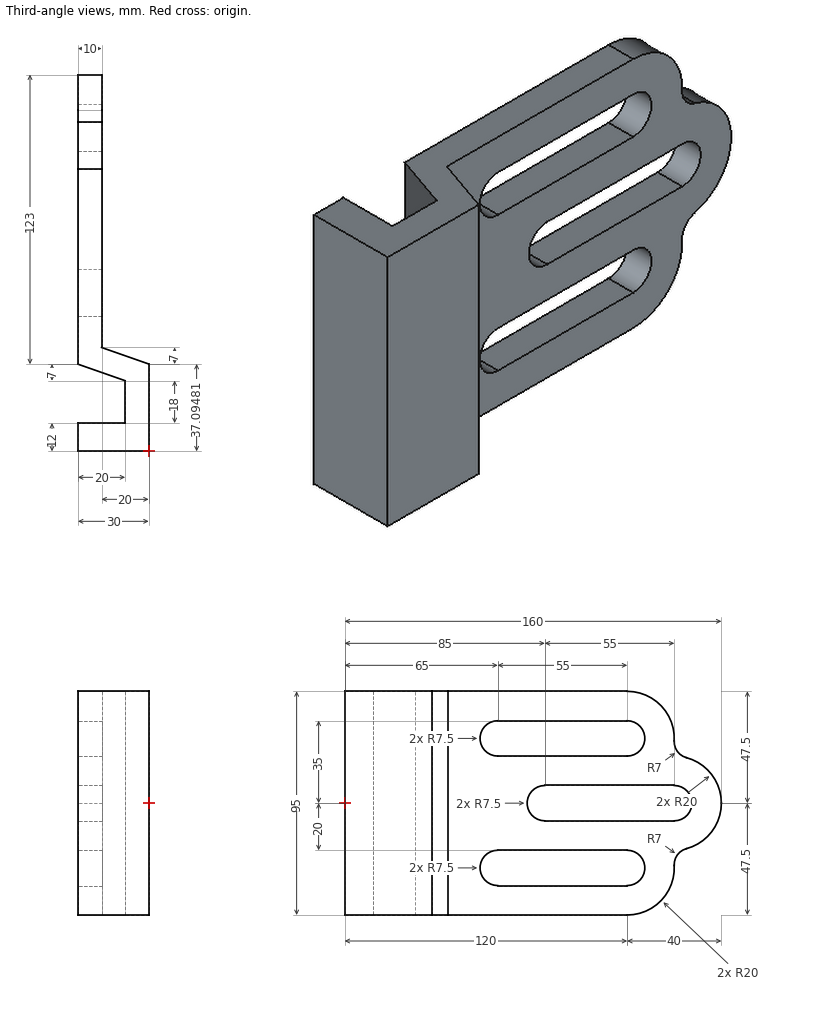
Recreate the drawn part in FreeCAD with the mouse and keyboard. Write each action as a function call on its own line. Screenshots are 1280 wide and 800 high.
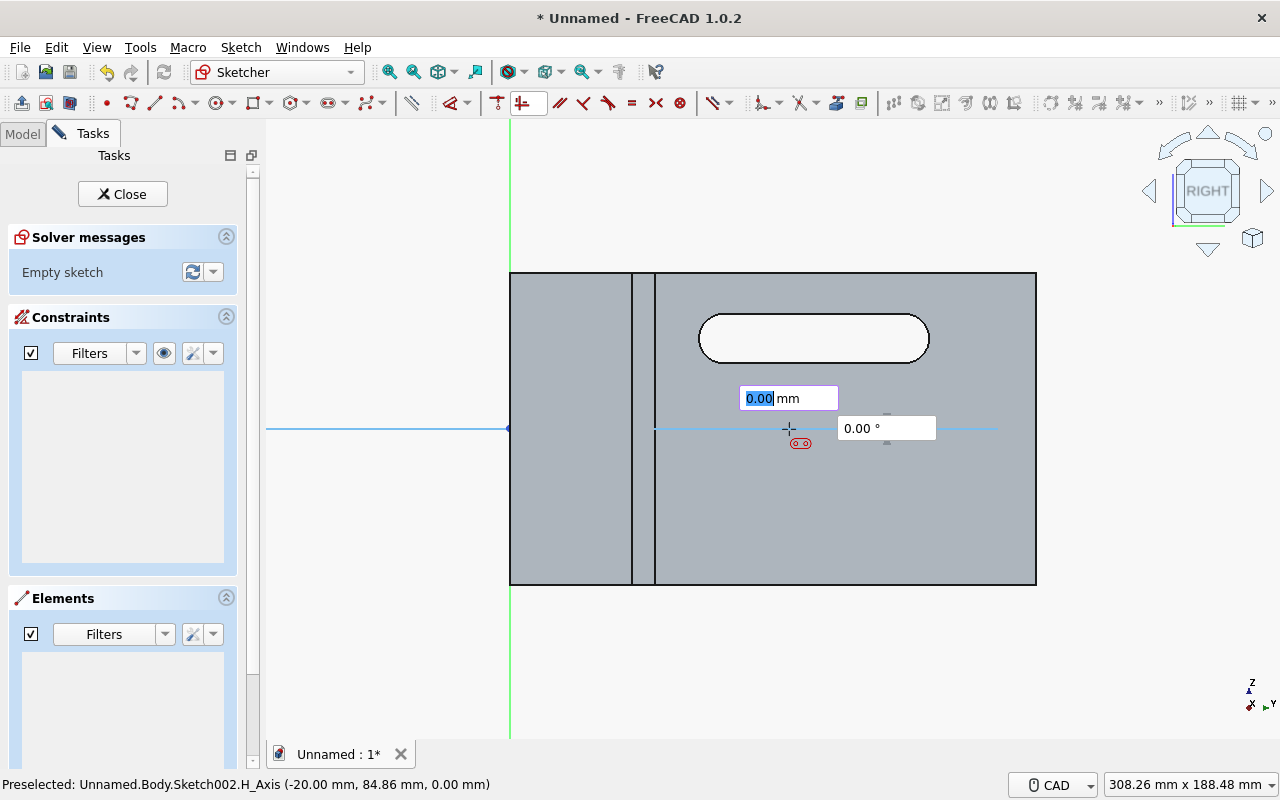
click(970, 420)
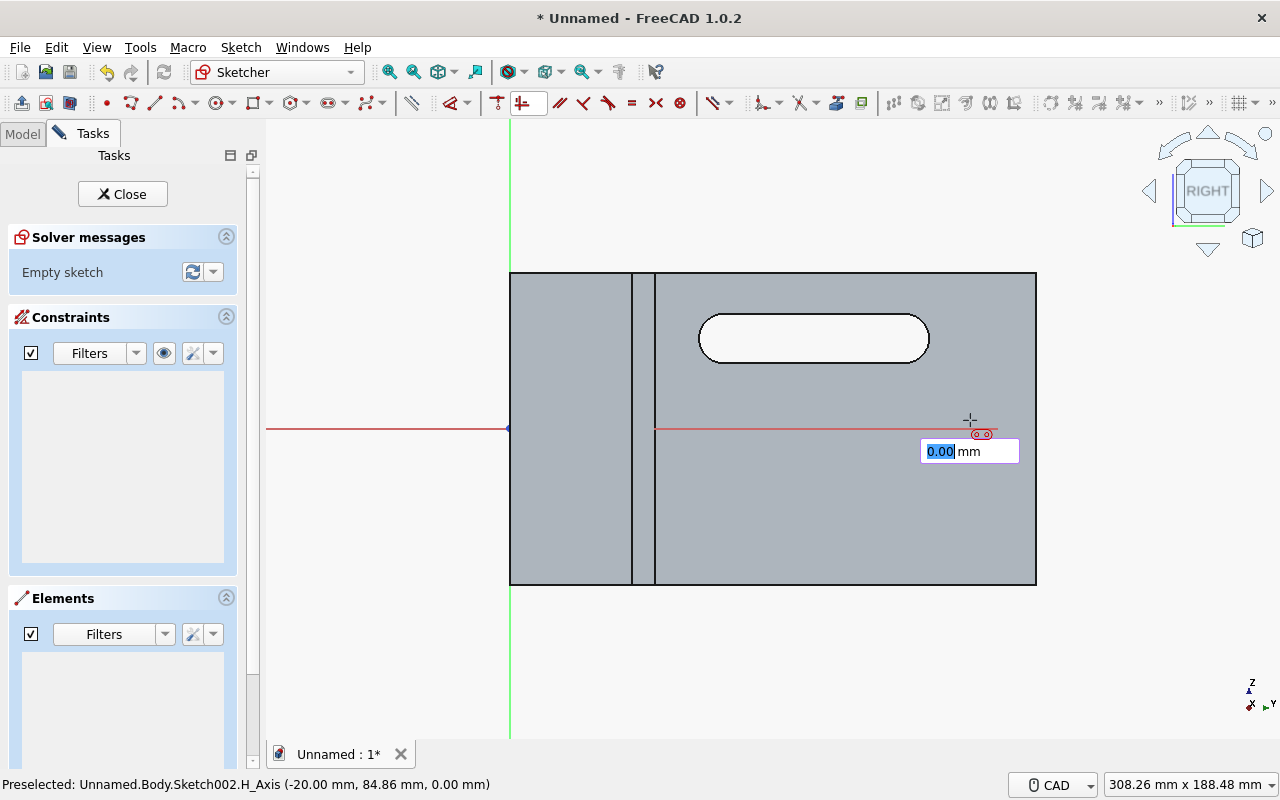
click(880, 404)
key(Escape)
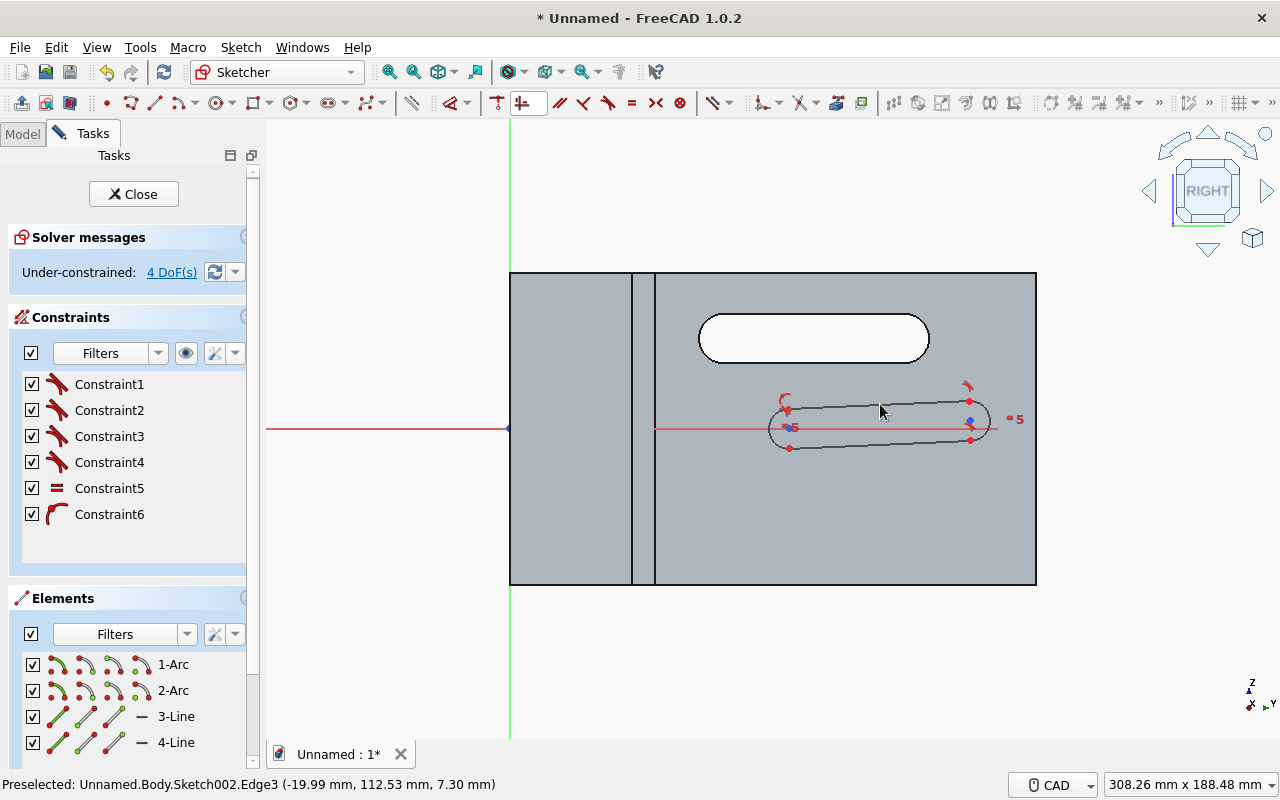
click(842, 407)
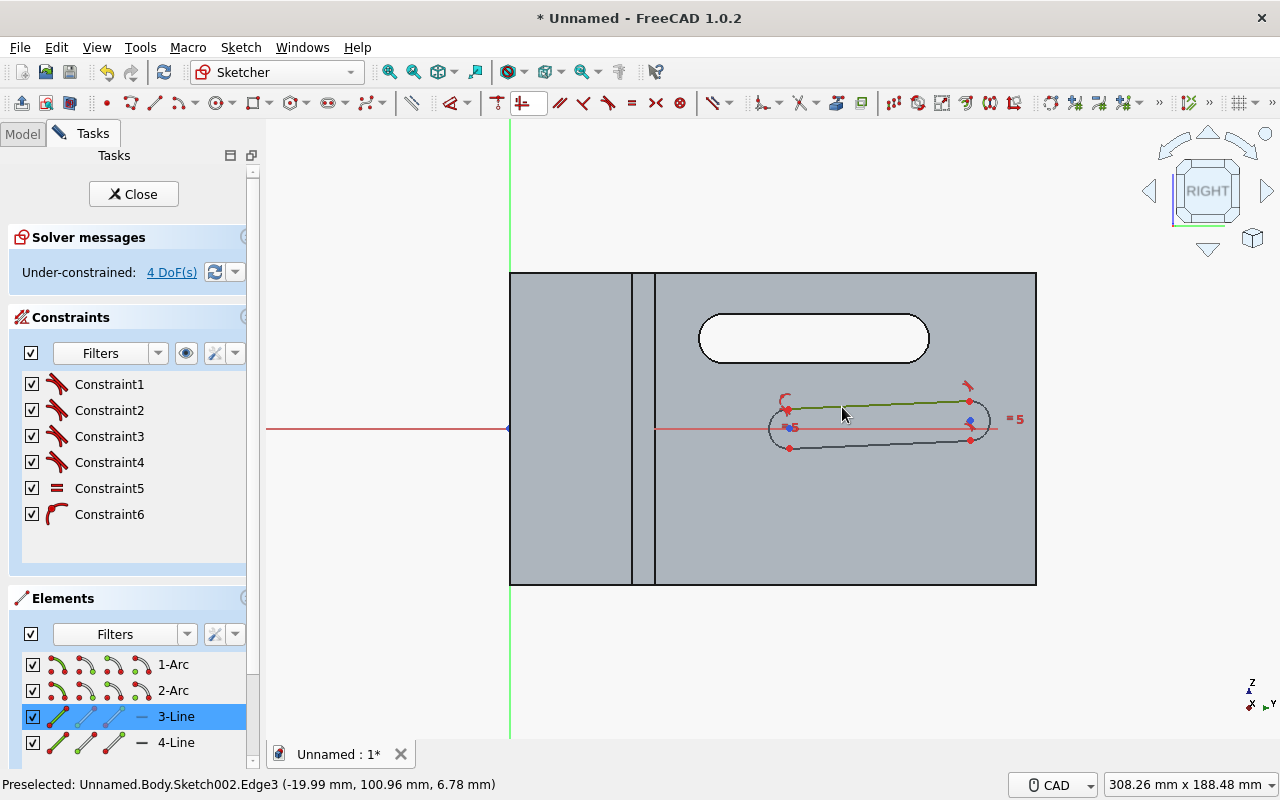
click(542, 104)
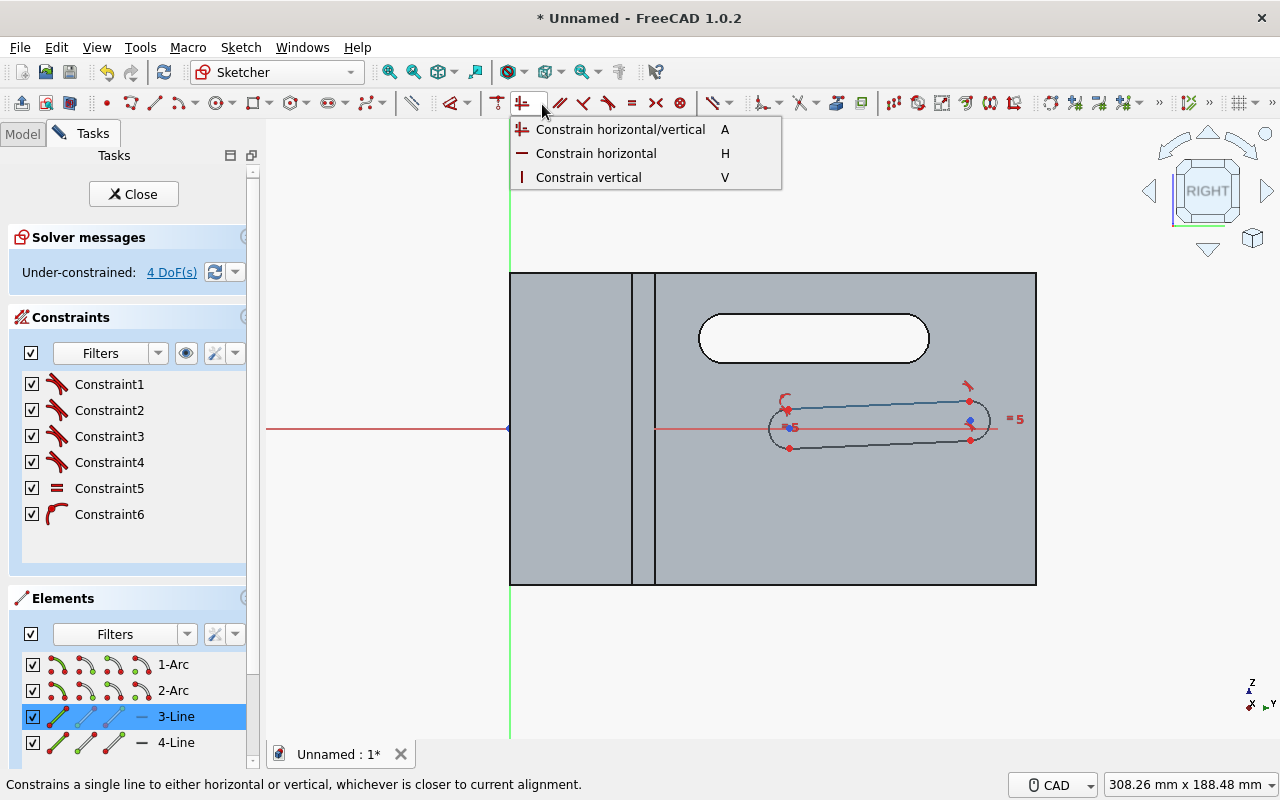
click(646, 153)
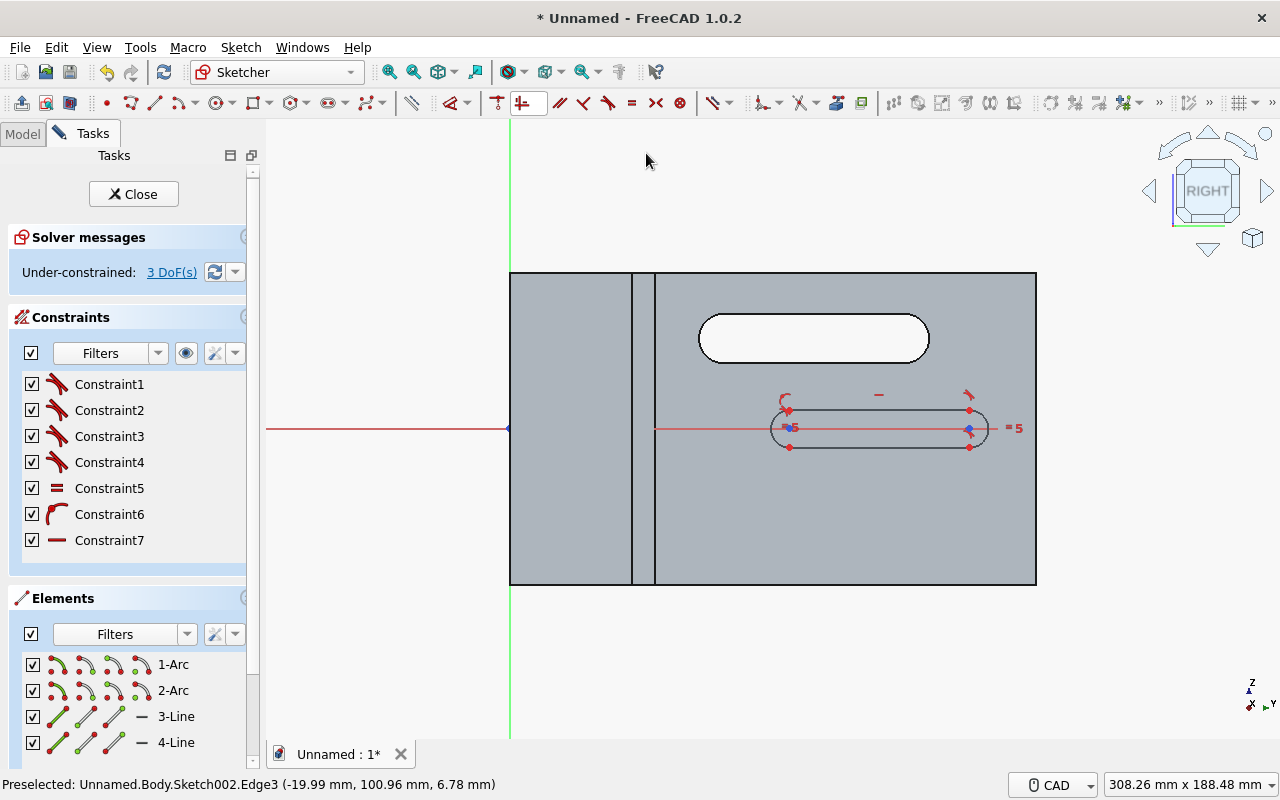
click(450, 104)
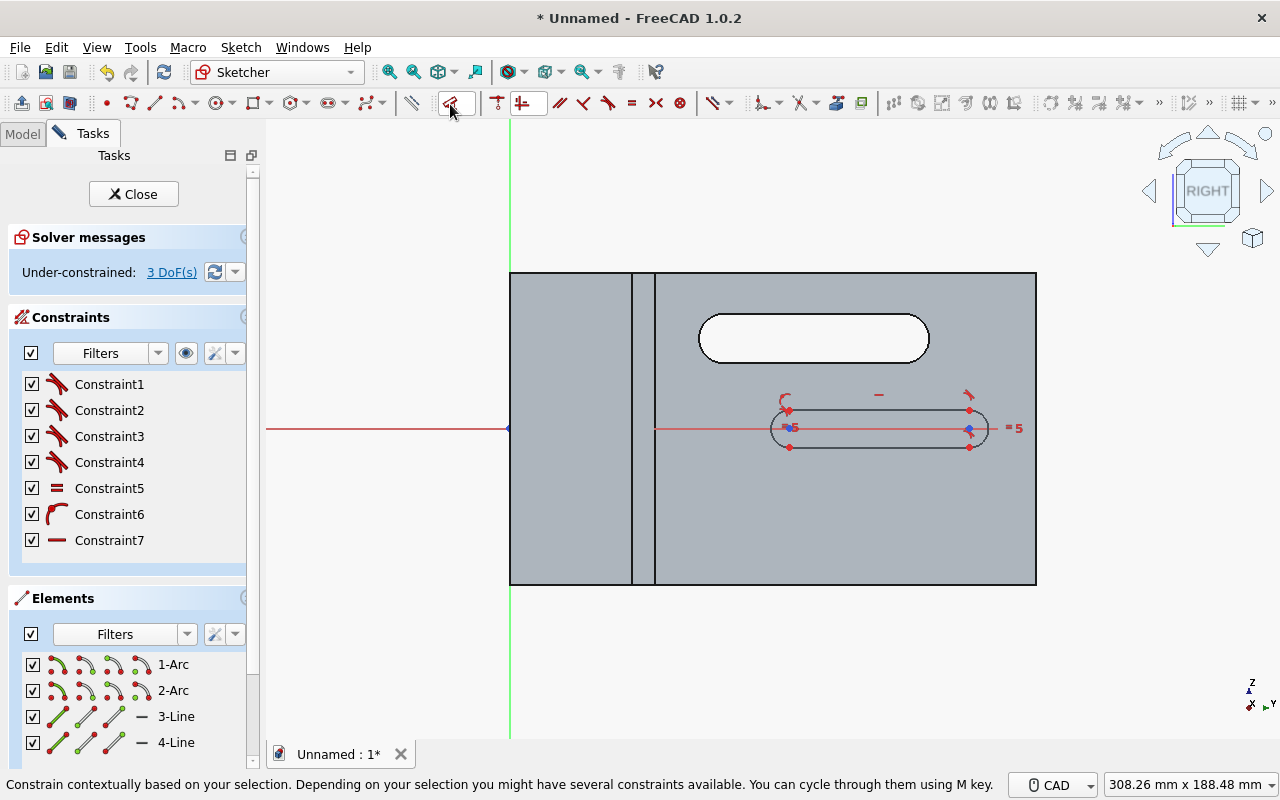
scroll(775, 418, up, 3)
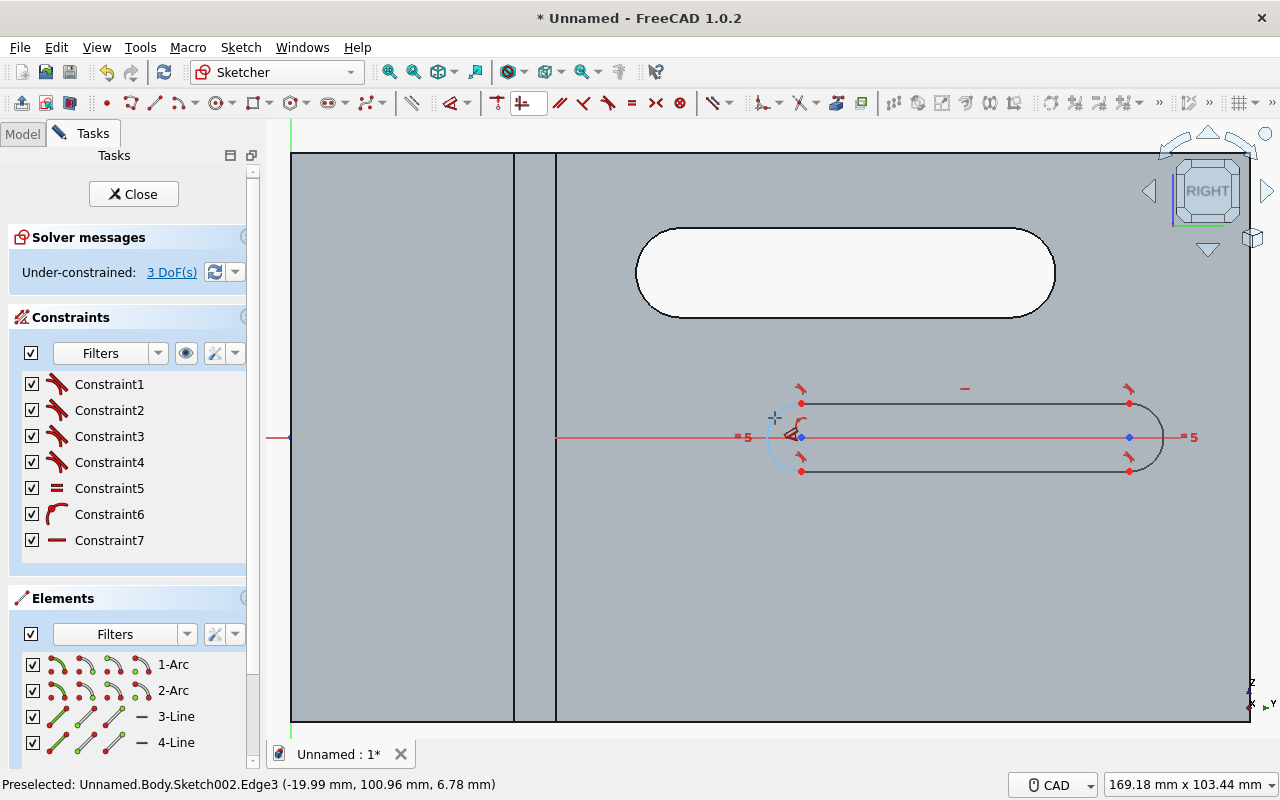
click(774, 418)
click(748, 399)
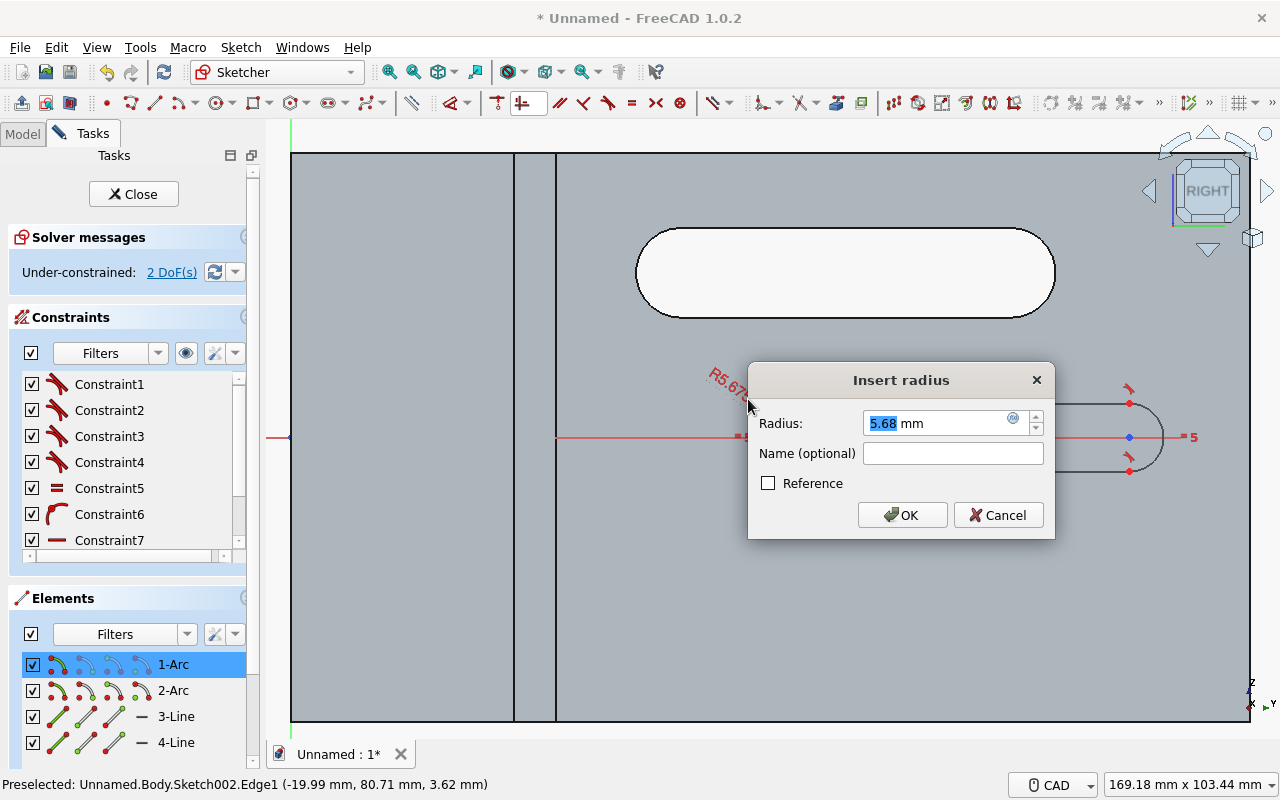
text(7.5)
key(Return)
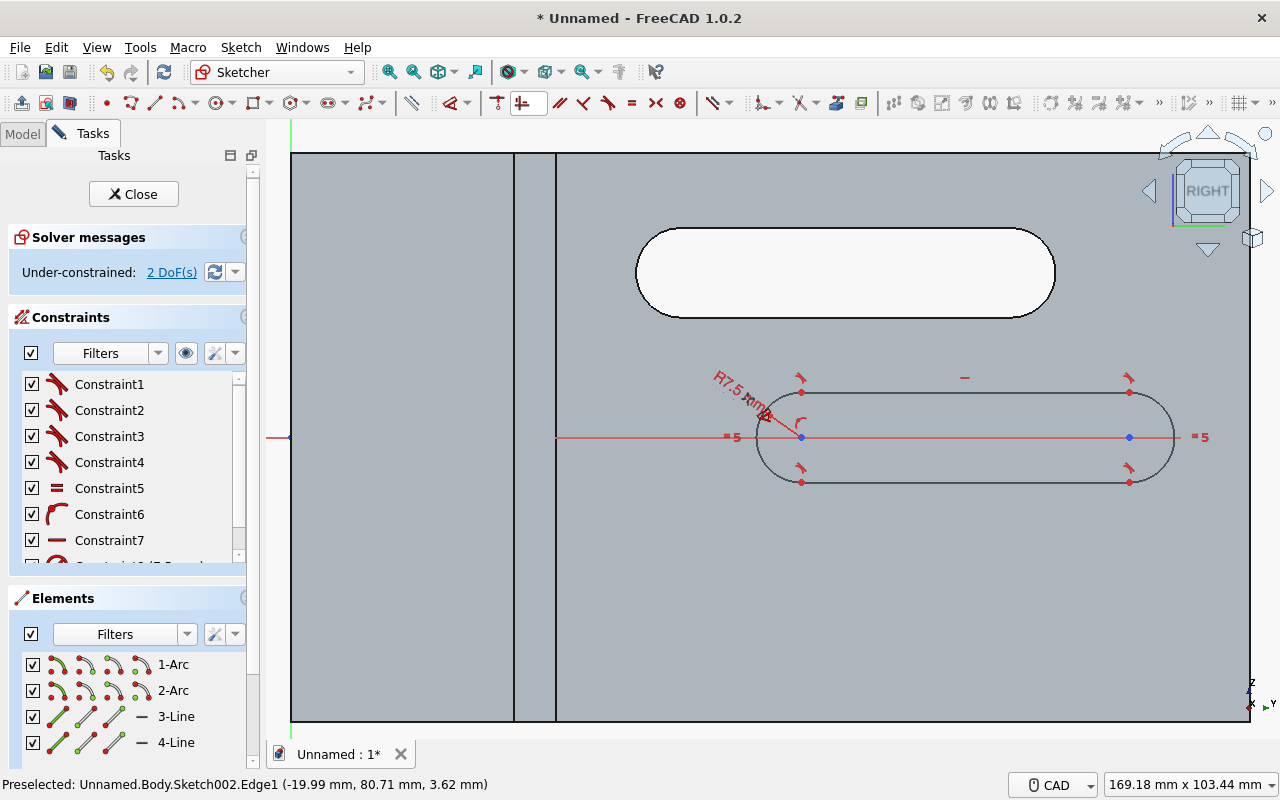
click(900, 393)
click(958, 359)